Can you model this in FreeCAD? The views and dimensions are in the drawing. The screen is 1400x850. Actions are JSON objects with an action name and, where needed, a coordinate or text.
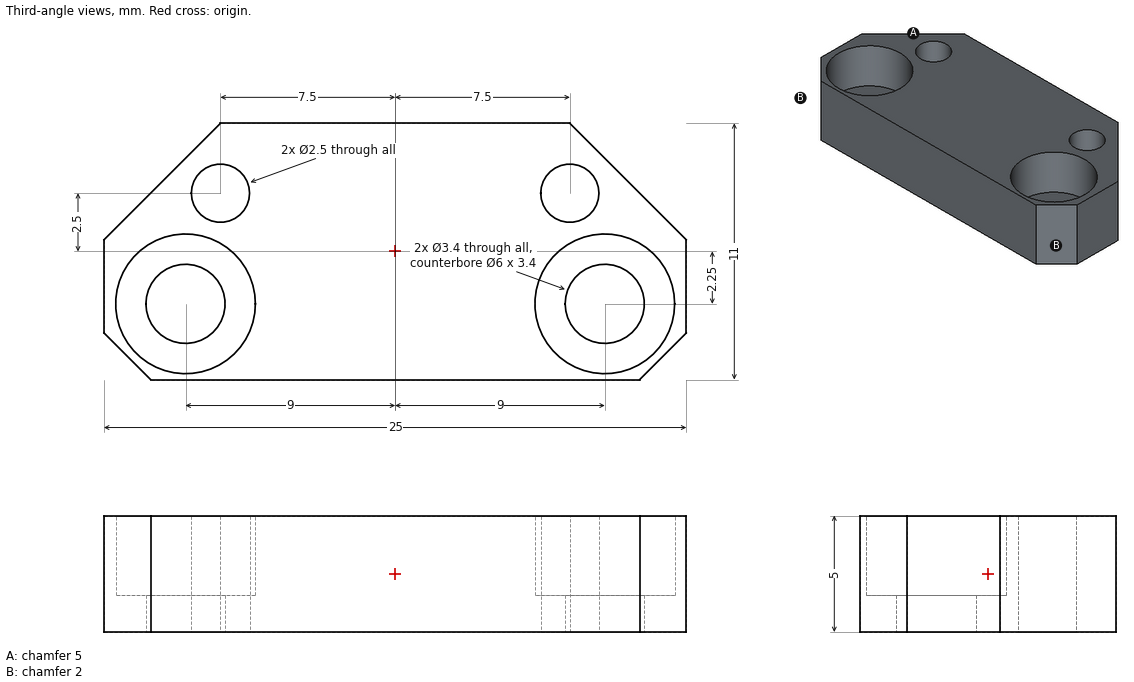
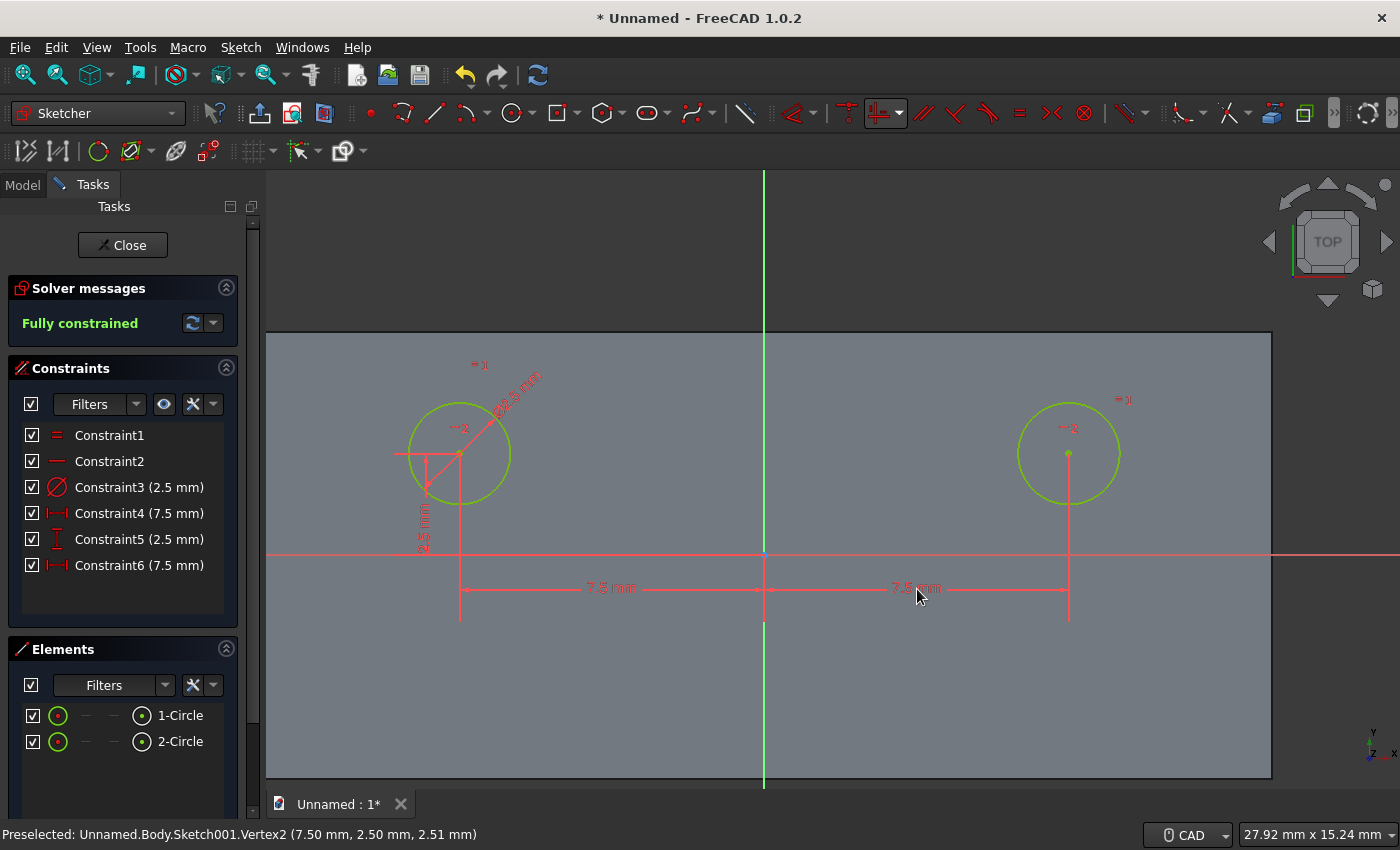
{"action": "left_click", "coordinate": [123, 245]}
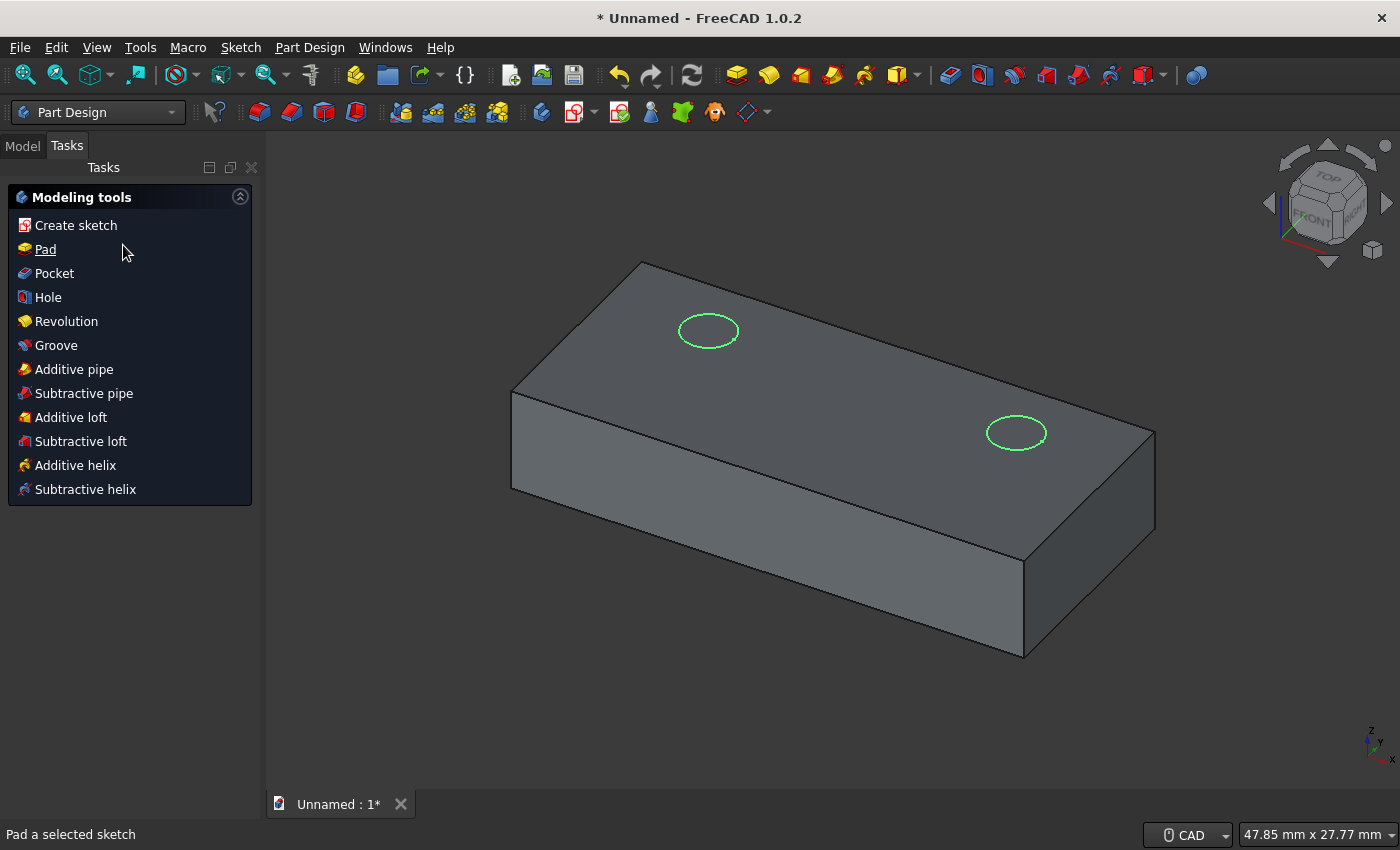
{"action": "left_click", "coordinate": [984, 76]}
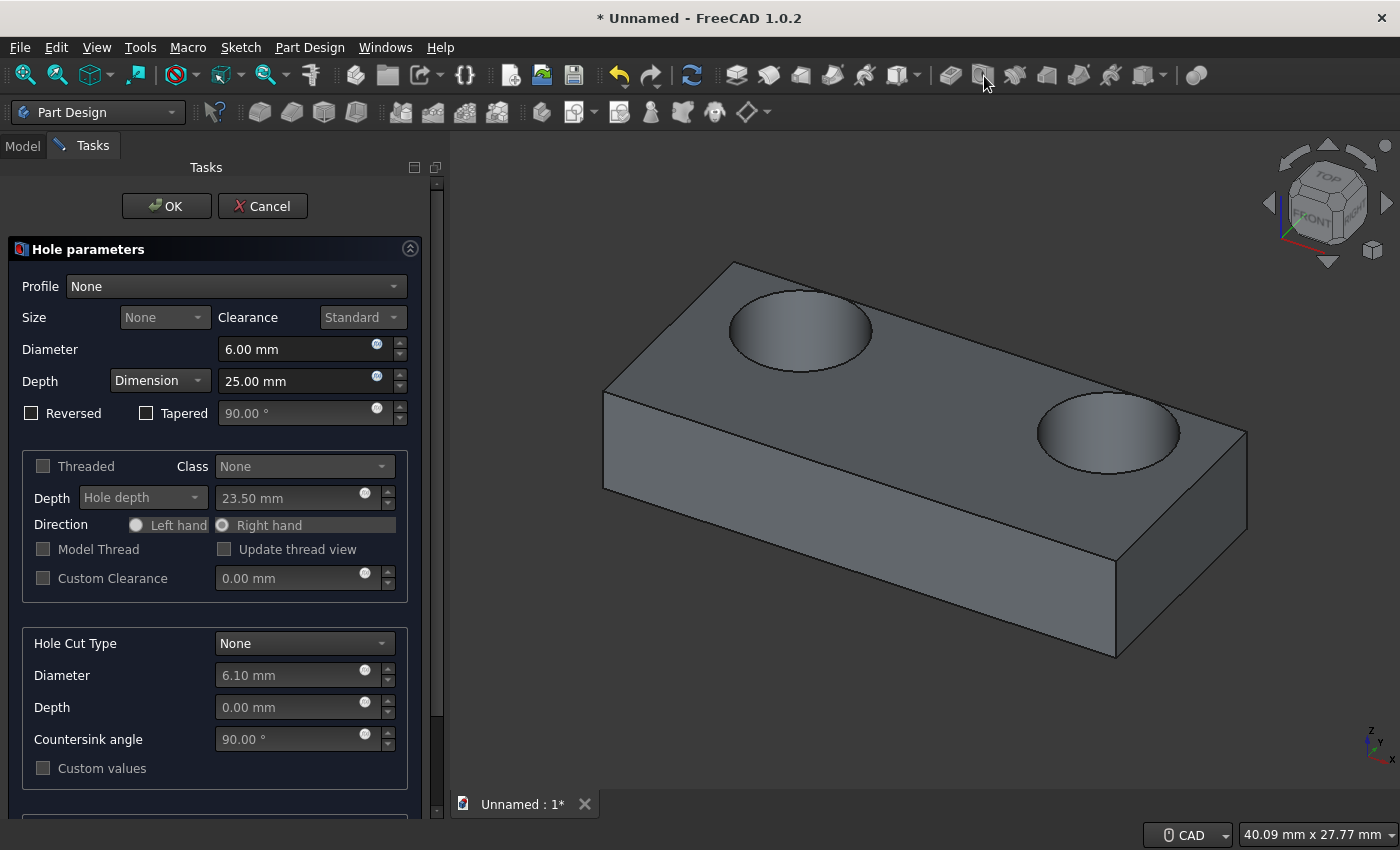
{"action": "triple_click", "coordinate": [305, 349]}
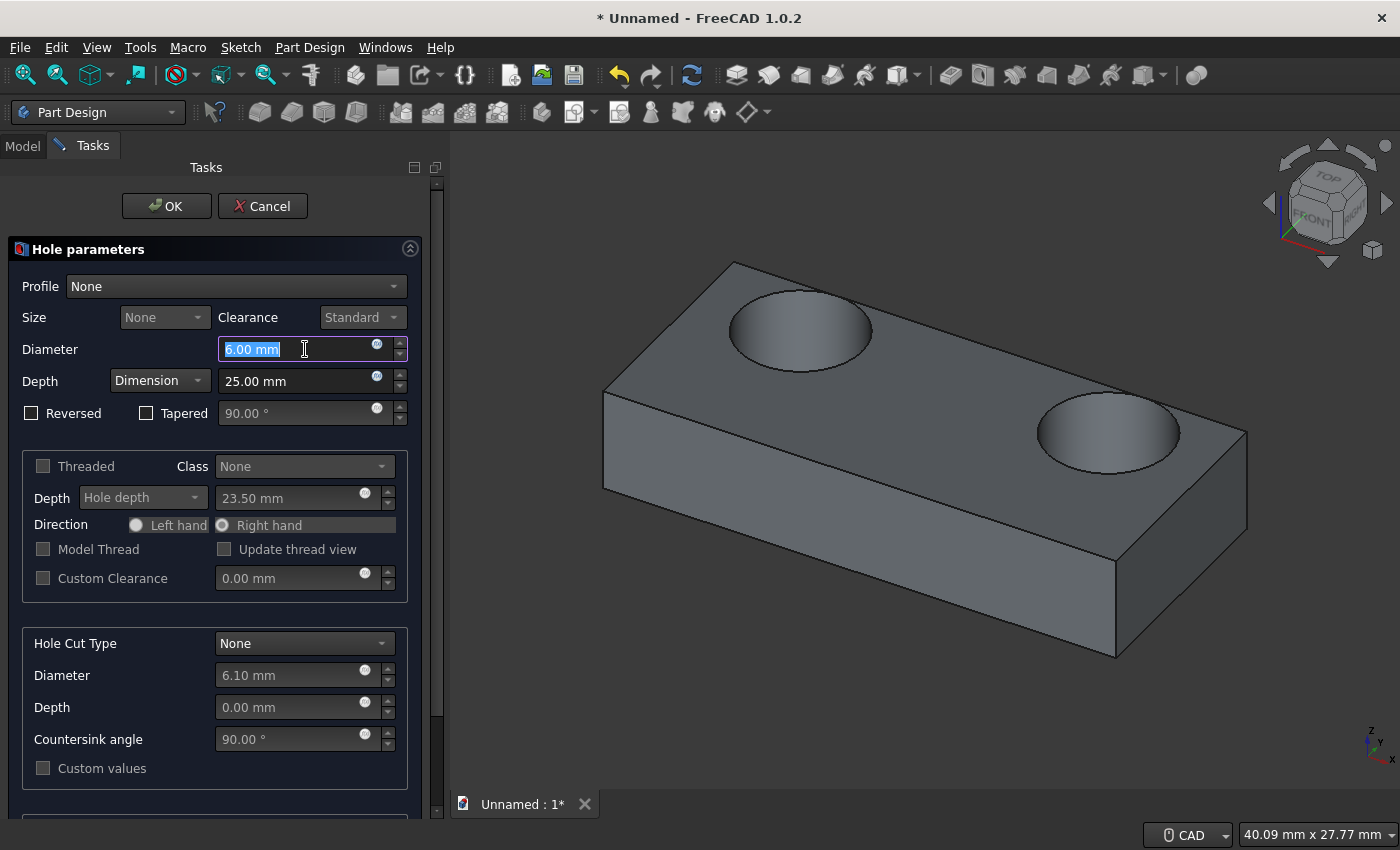
{"action": "type", "text": "2.5"}
{"action": "key", "text": "Tab"}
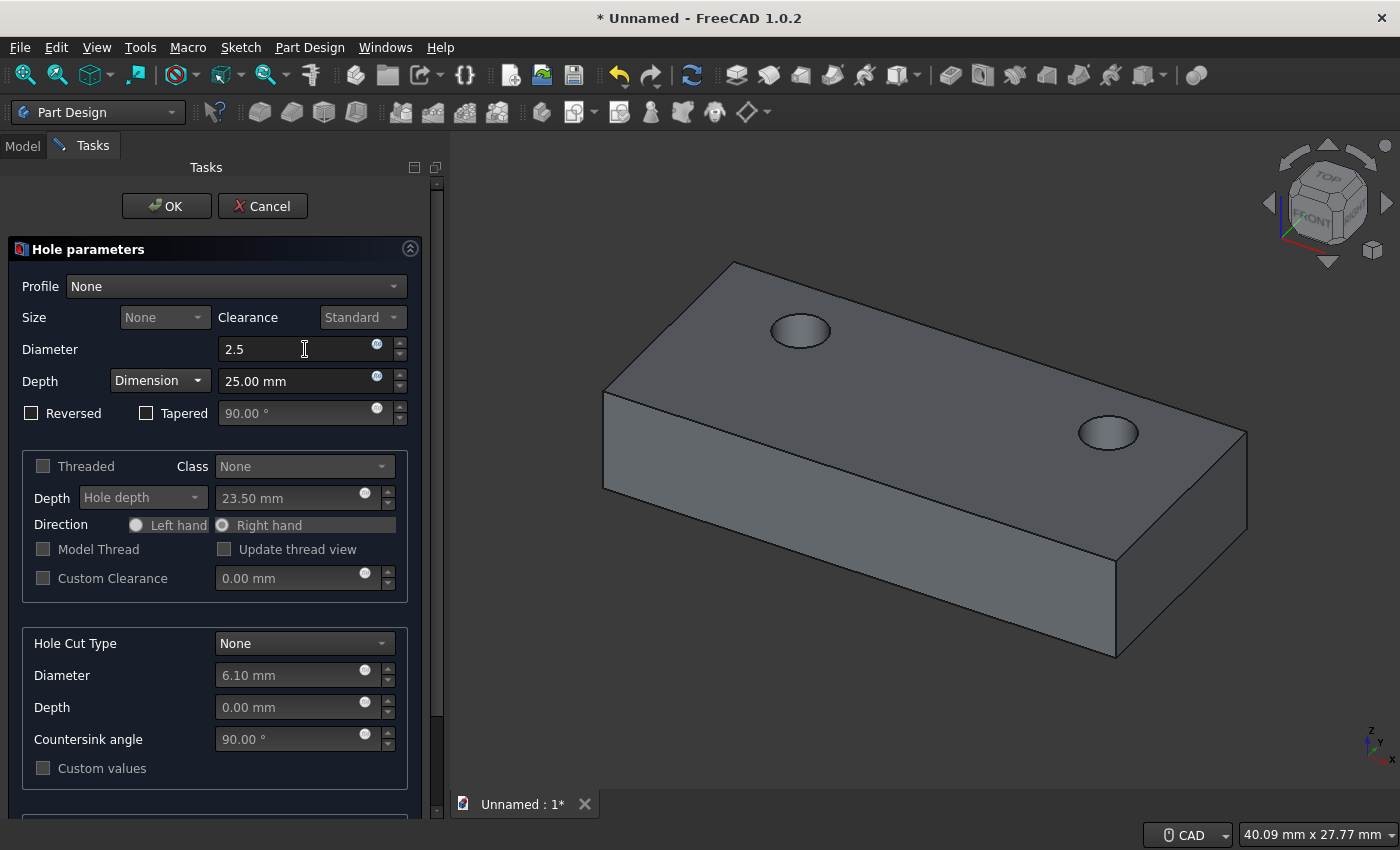
{"action": "left_click", "coordinate": [161, 380]}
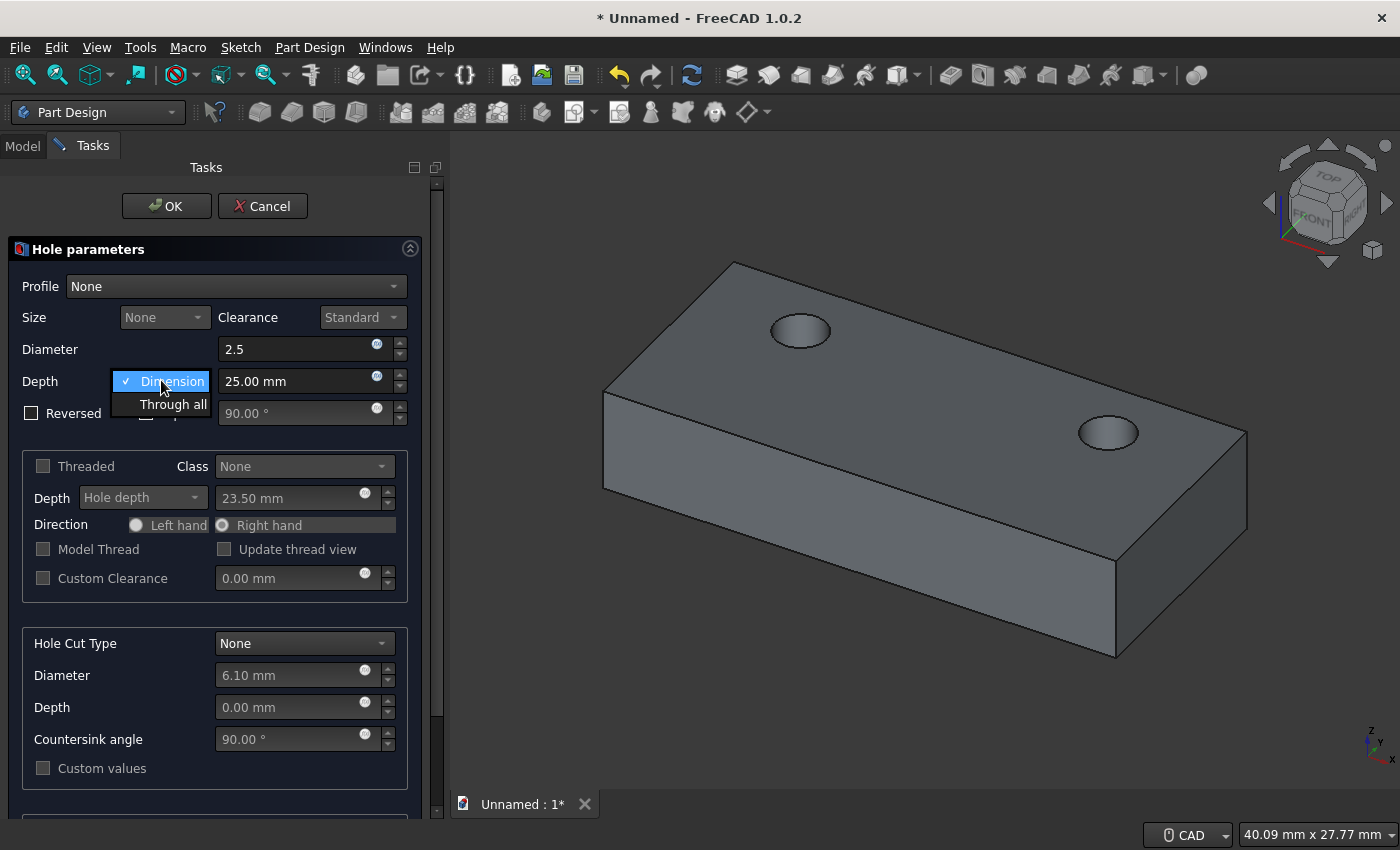
{"action": "left_click", "coordinate": [160, 404]}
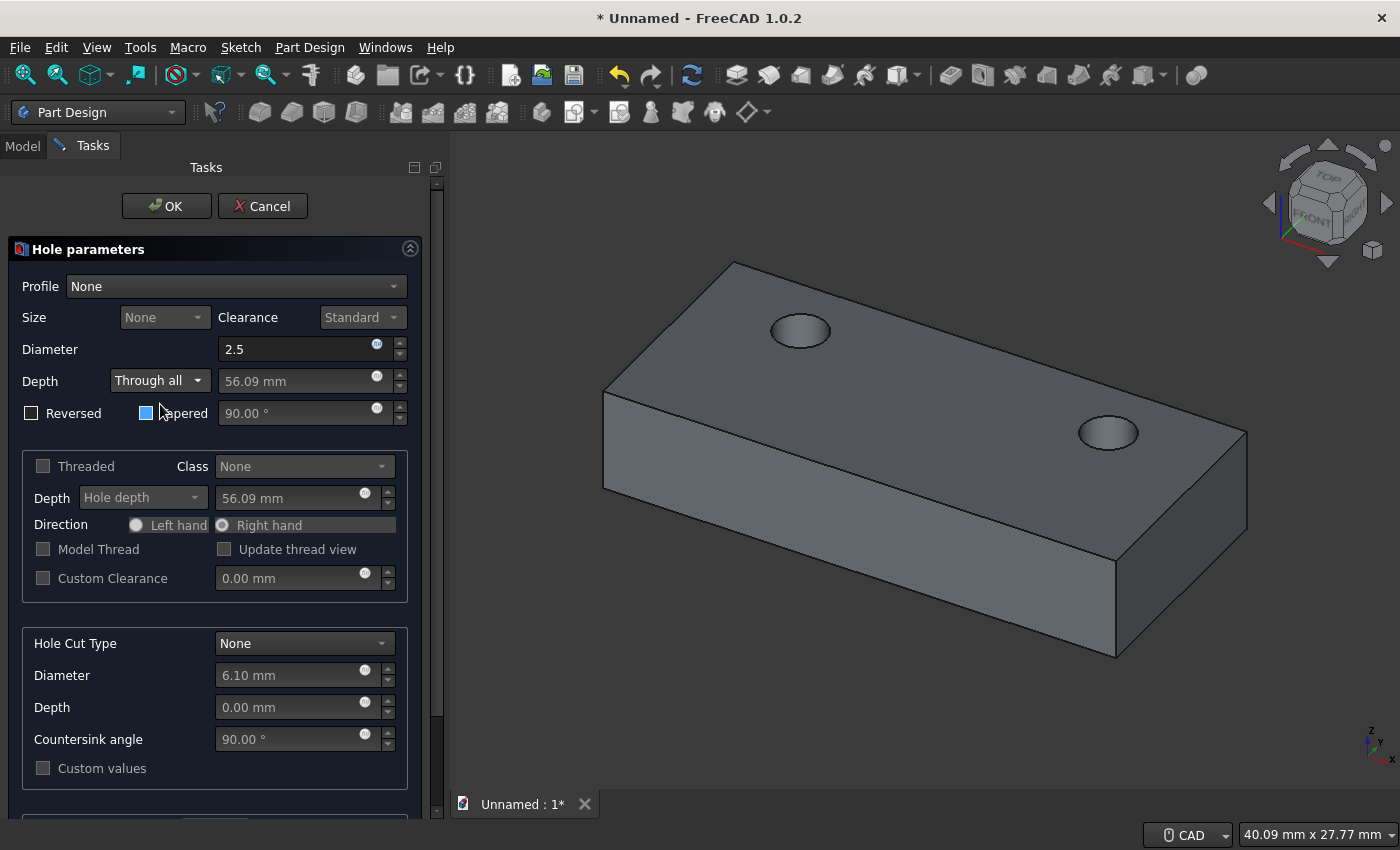
{"action": "left_click", "coordinate": [167, 206]}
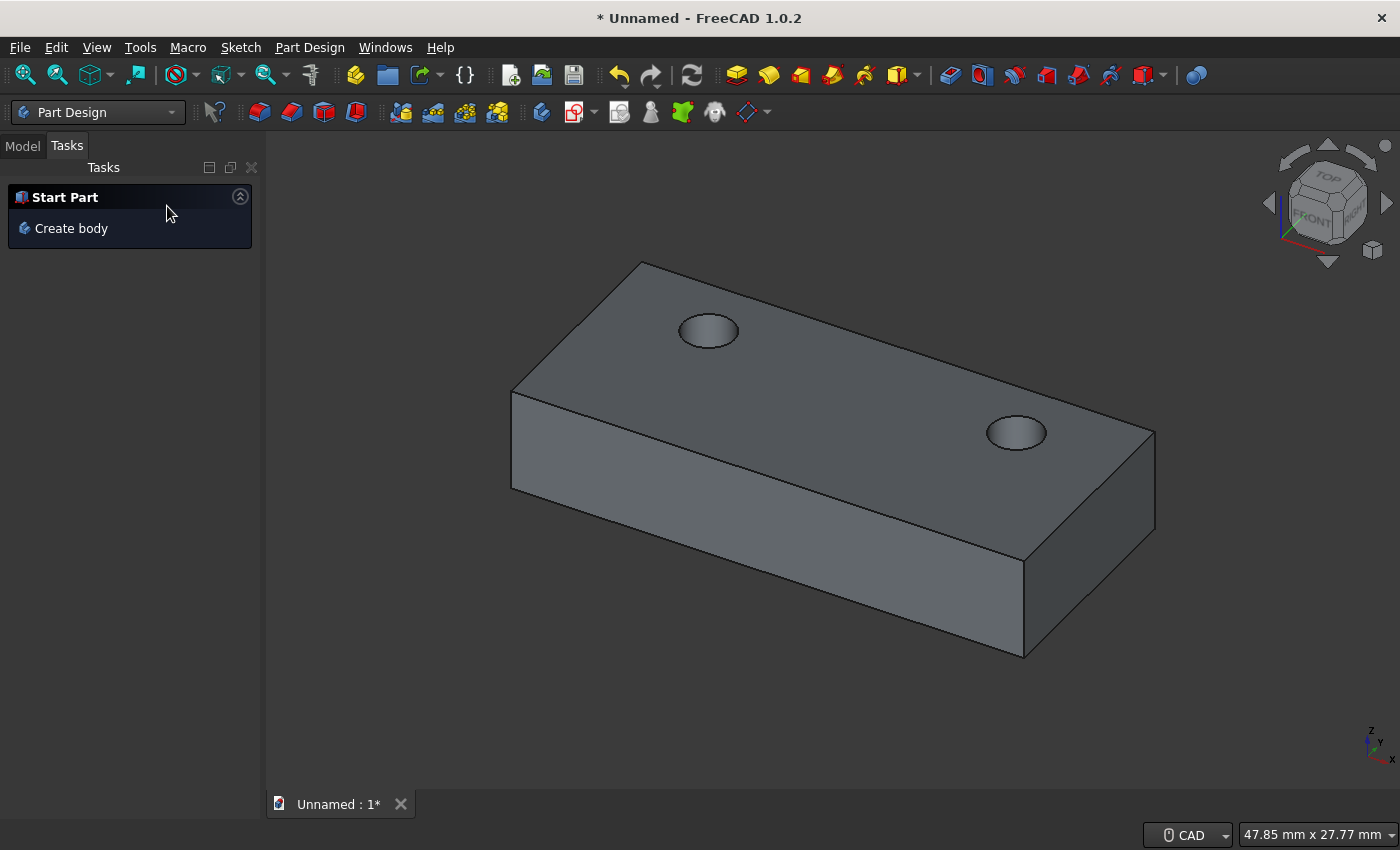
{"action": "left_click", "coordinate": [833, 410]}